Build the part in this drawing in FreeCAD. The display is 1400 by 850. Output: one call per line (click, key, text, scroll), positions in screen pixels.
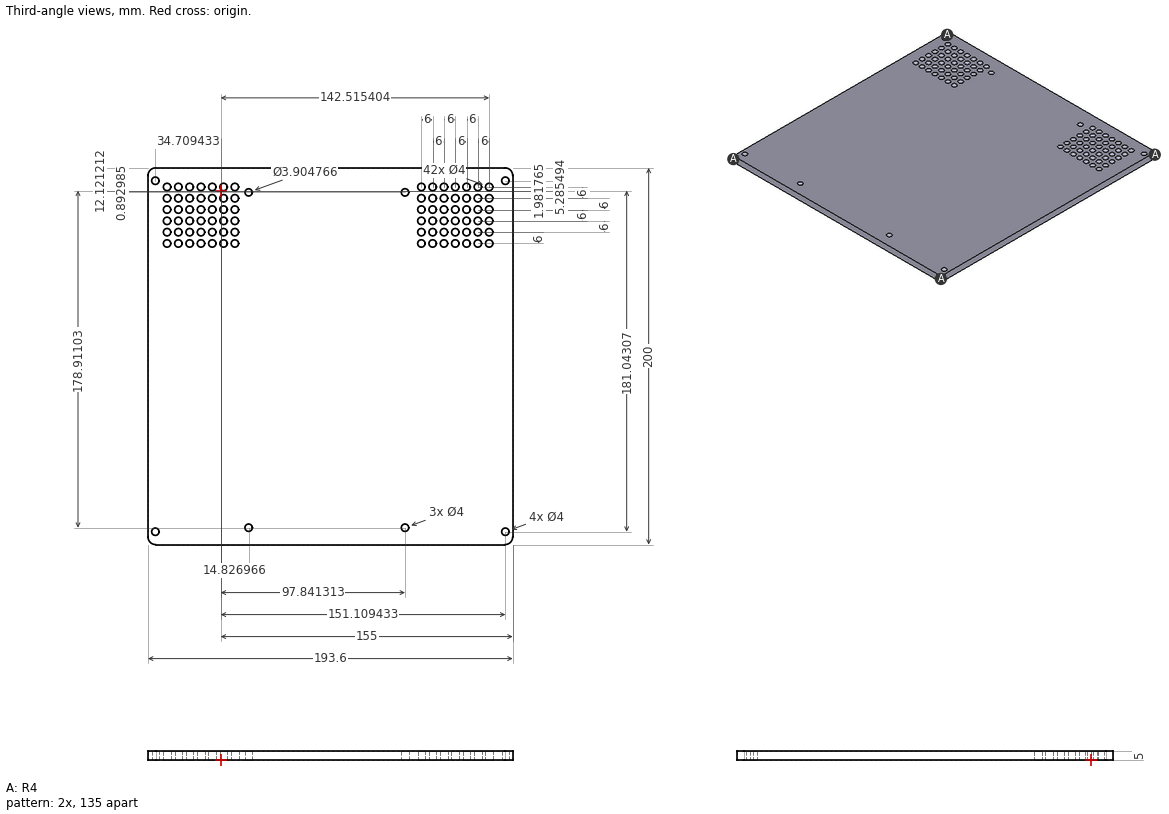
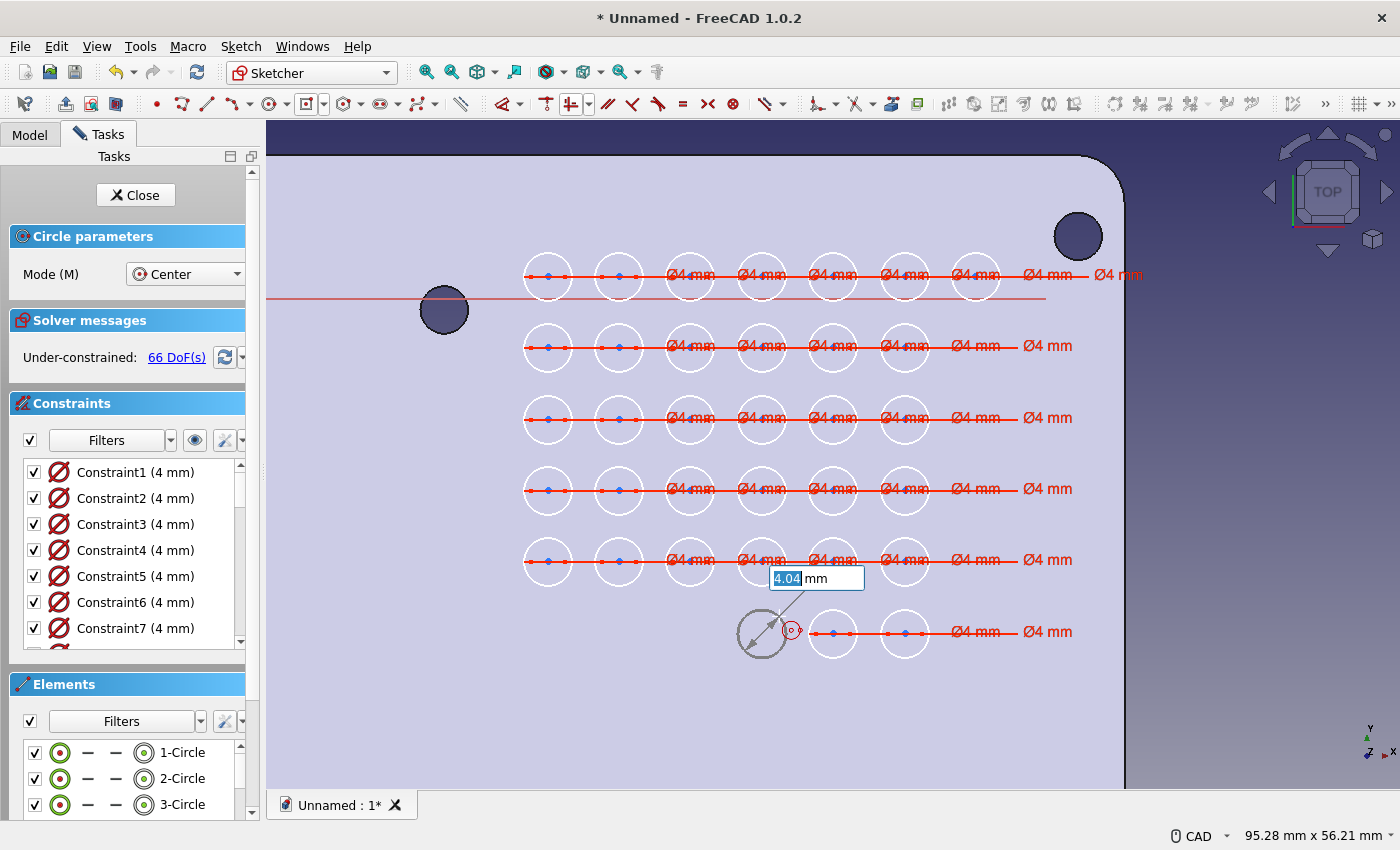
text(4)
key(Return)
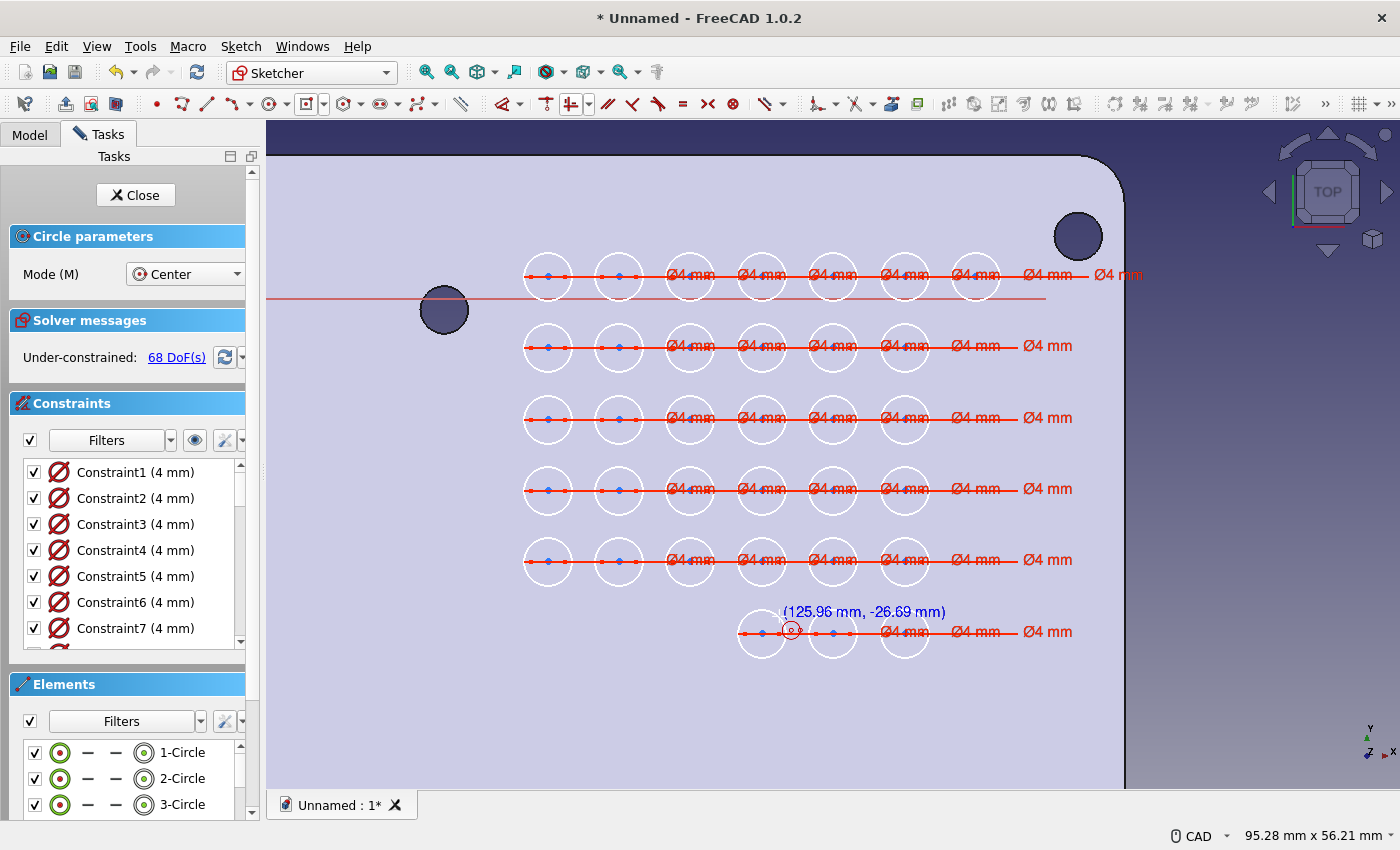
click(690, 633)
move(707, 616)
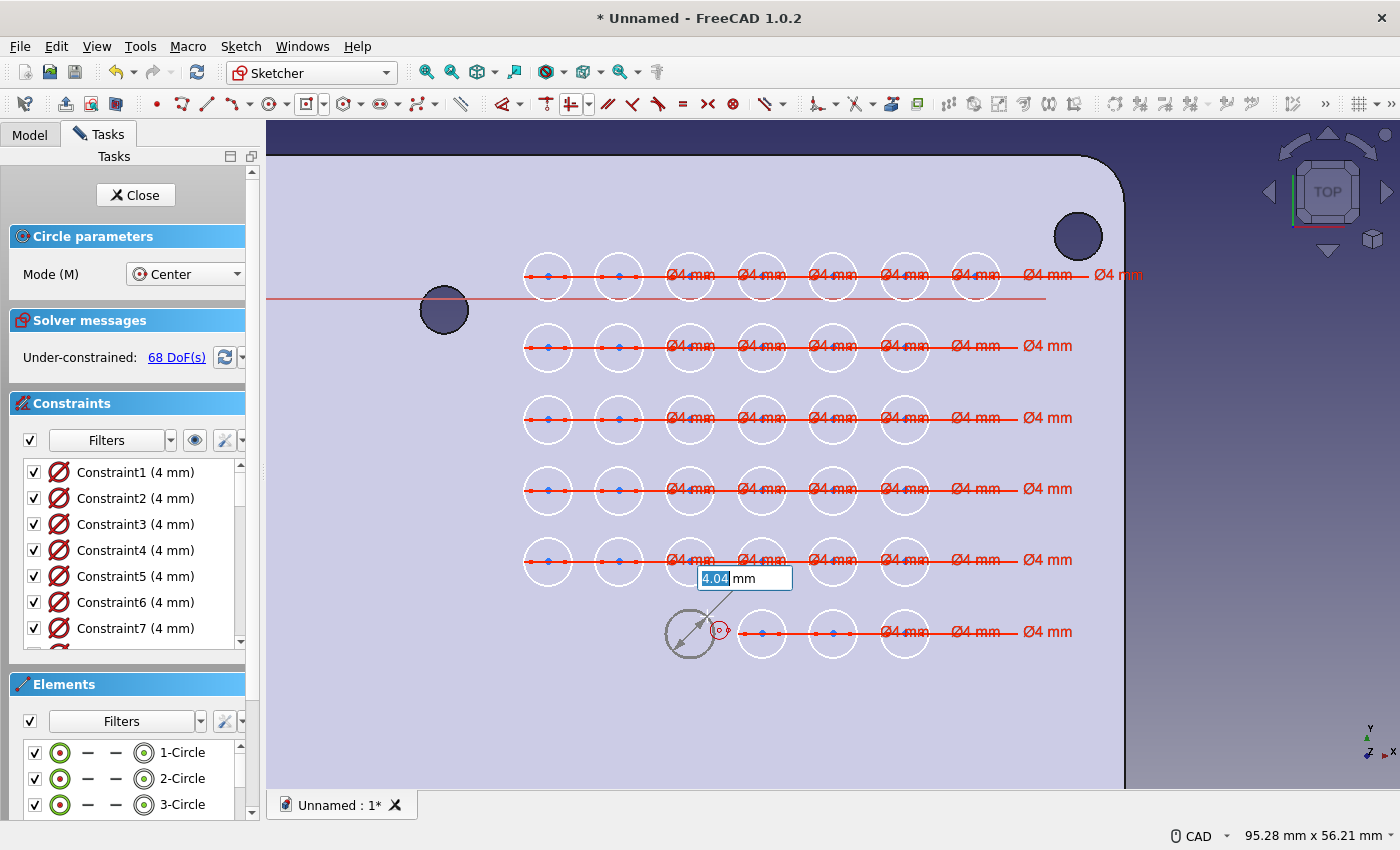
text(4)
key(Return)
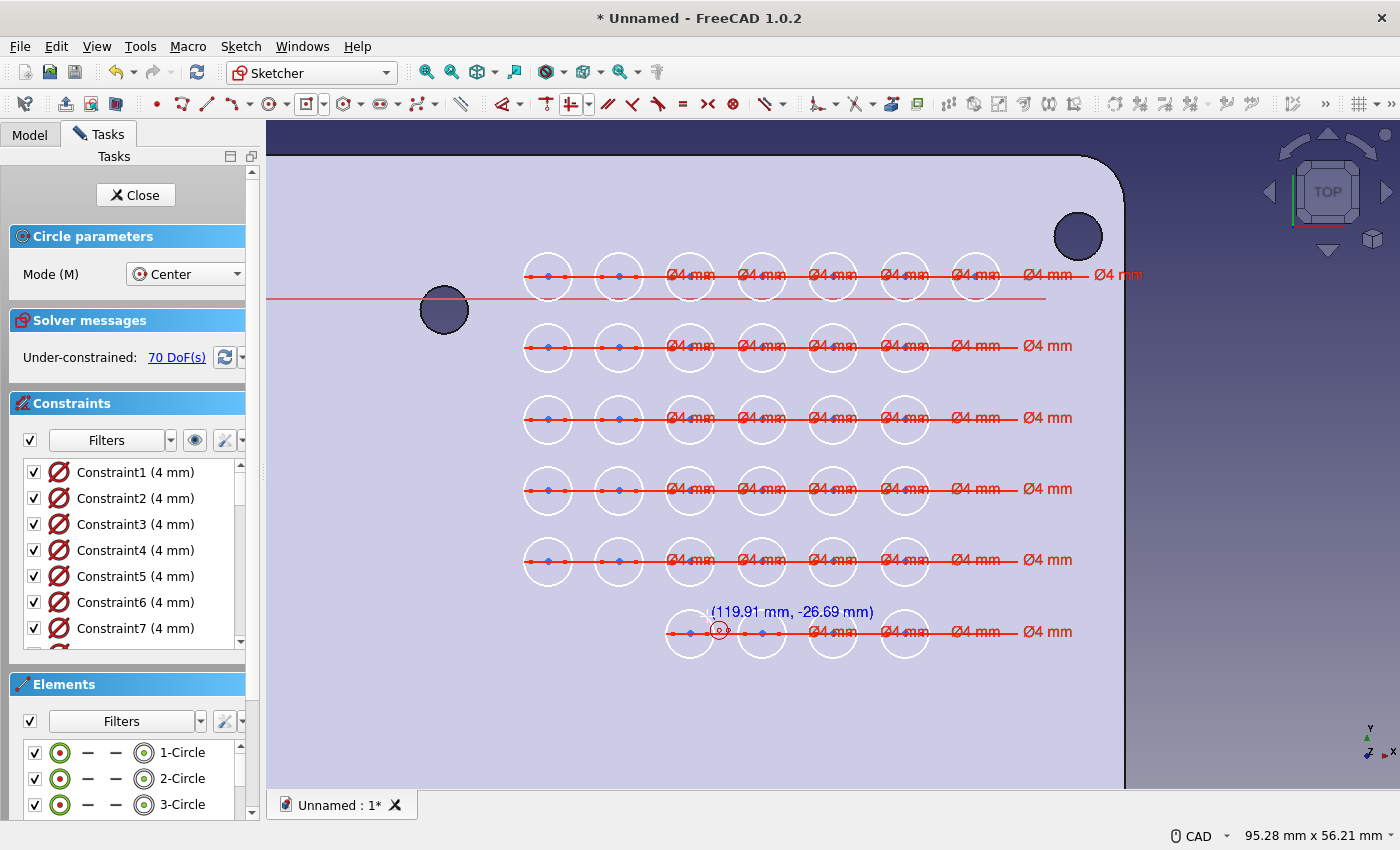
click(619, 633)
move(636, 616)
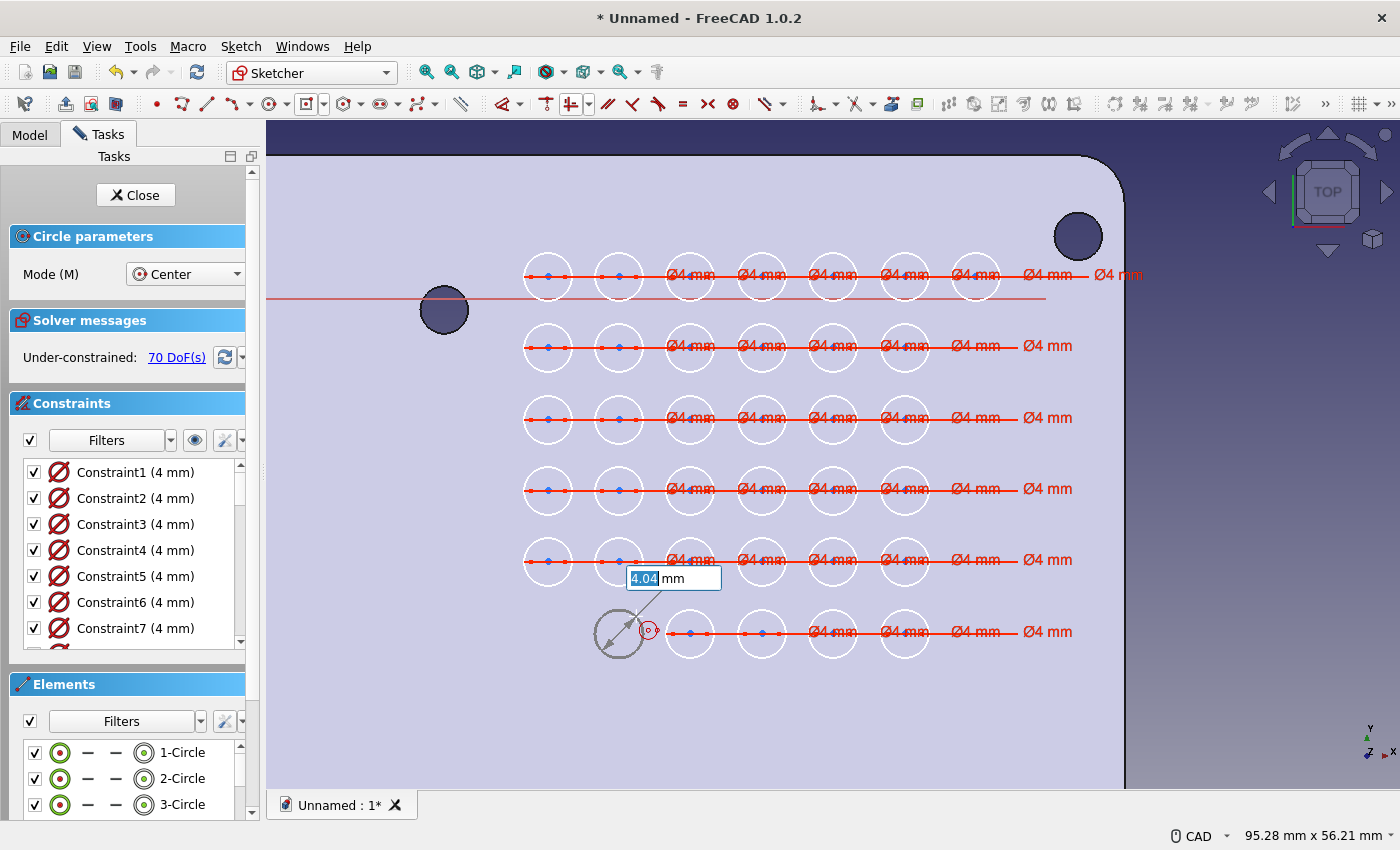
text(4)
key(Return)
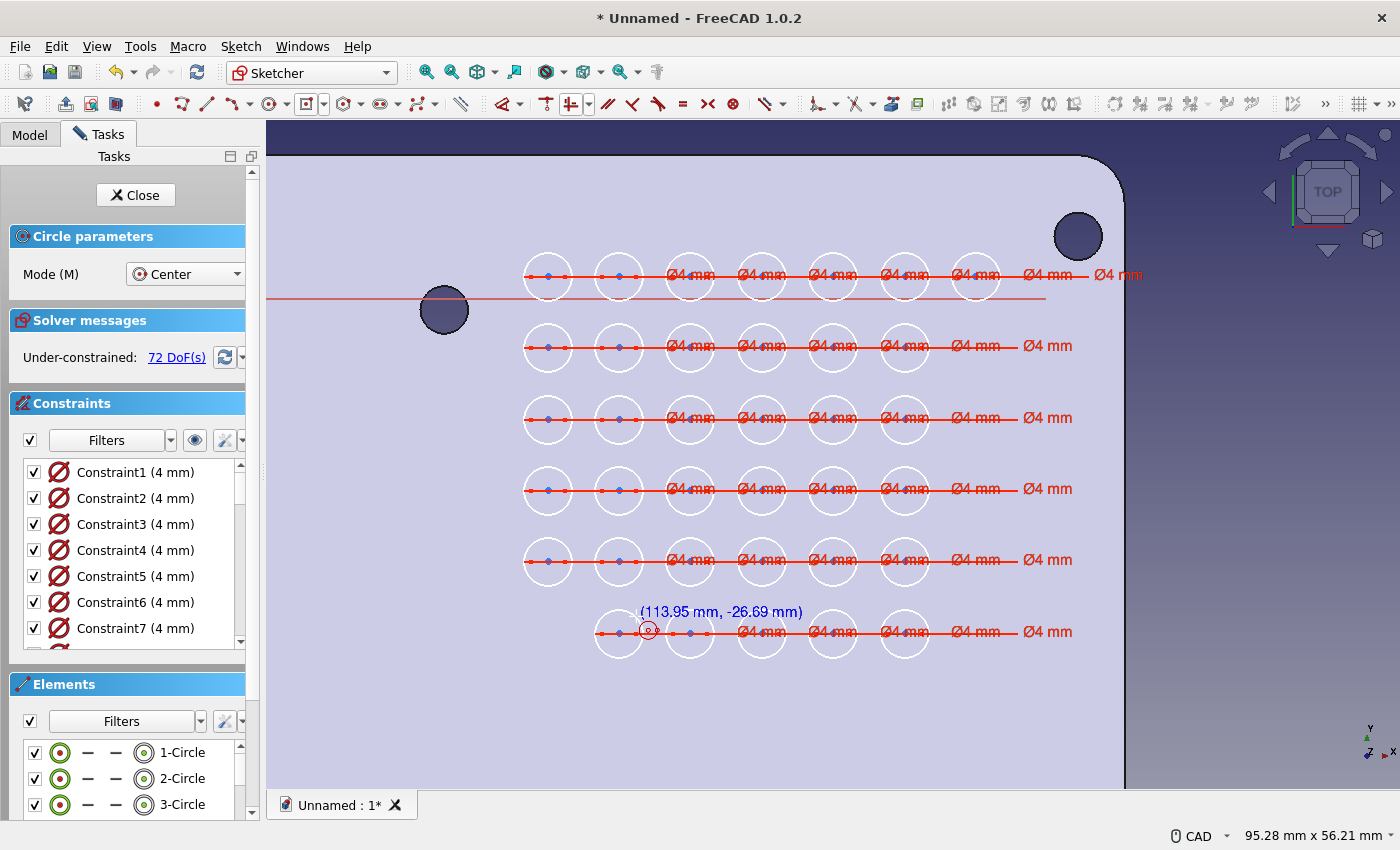
click(548, 633)
move(564, 616)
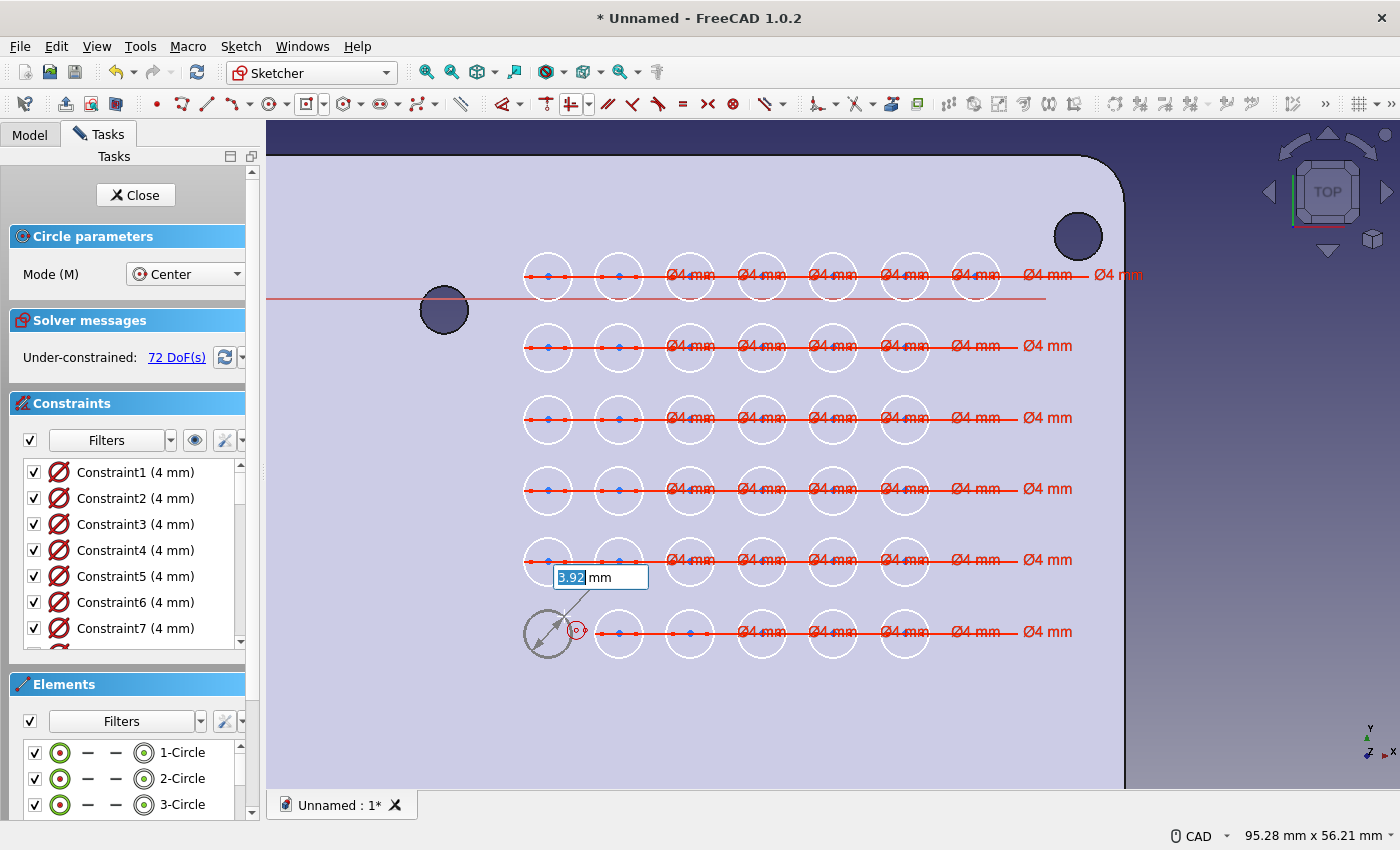
text(4)
key(Return)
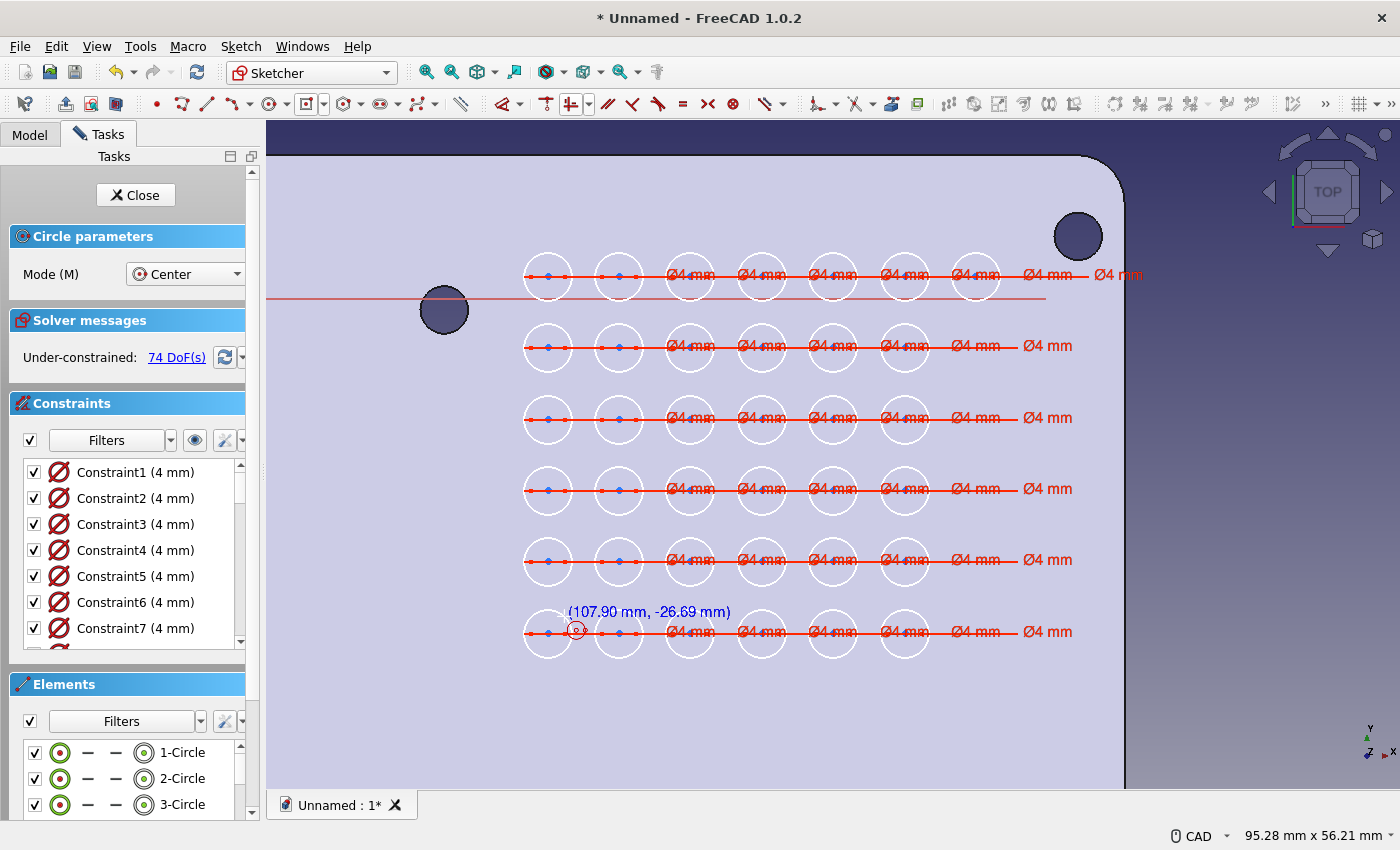
click(976, 347)
move(993, 330)